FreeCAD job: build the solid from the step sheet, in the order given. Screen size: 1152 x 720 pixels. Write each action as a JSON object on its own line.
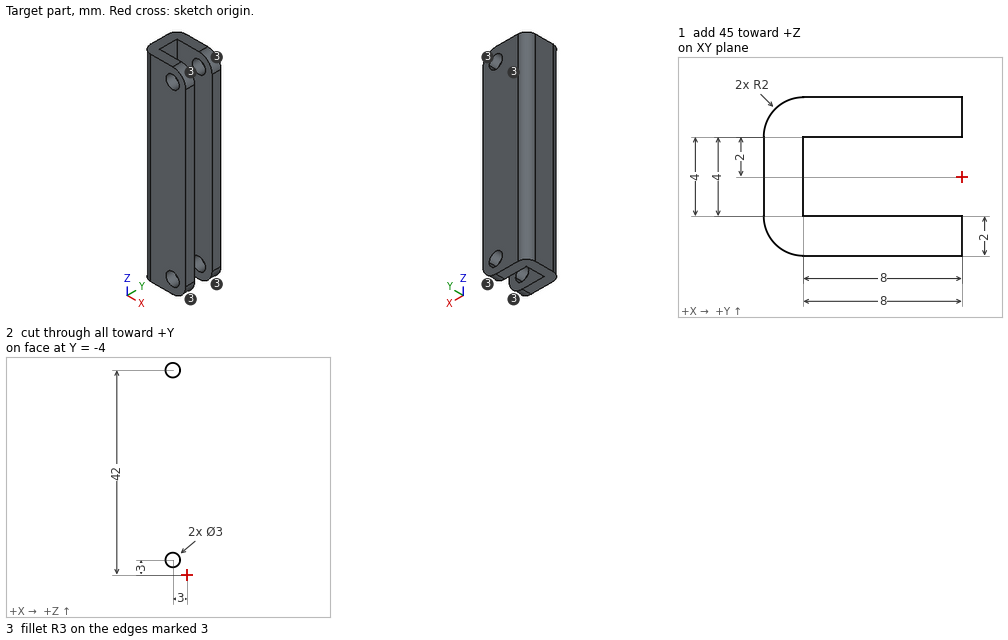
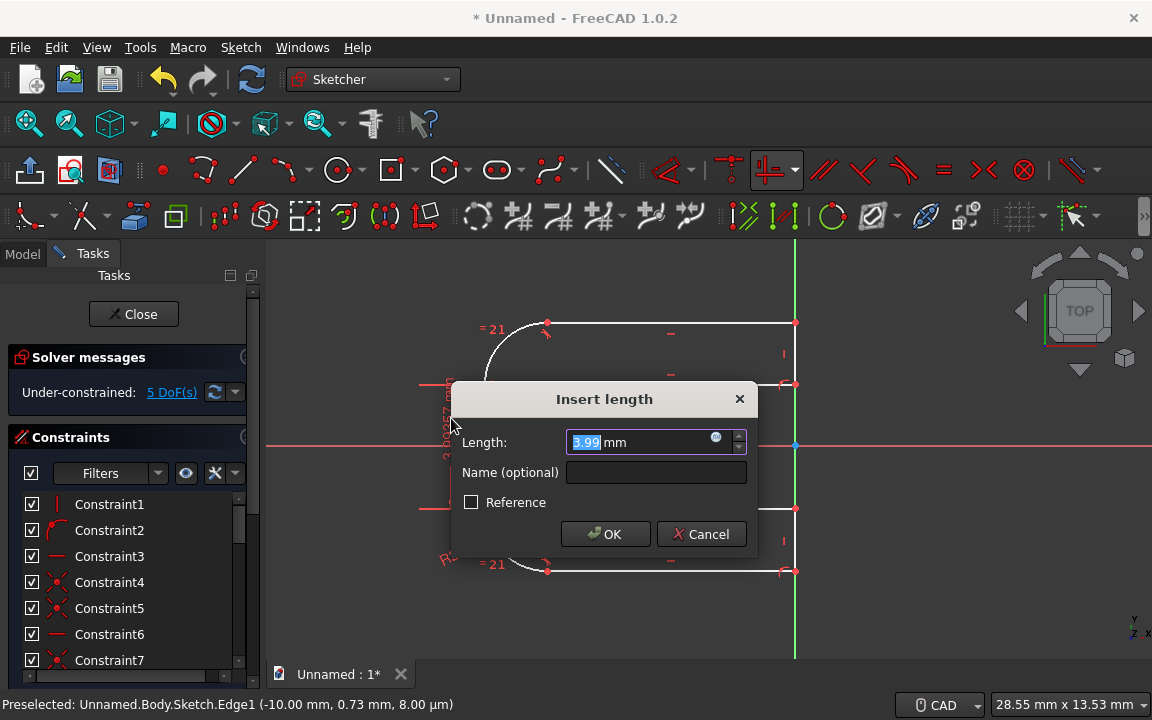
{"action": "type", "text": "4"}
{"action": "key", "text": "Return"}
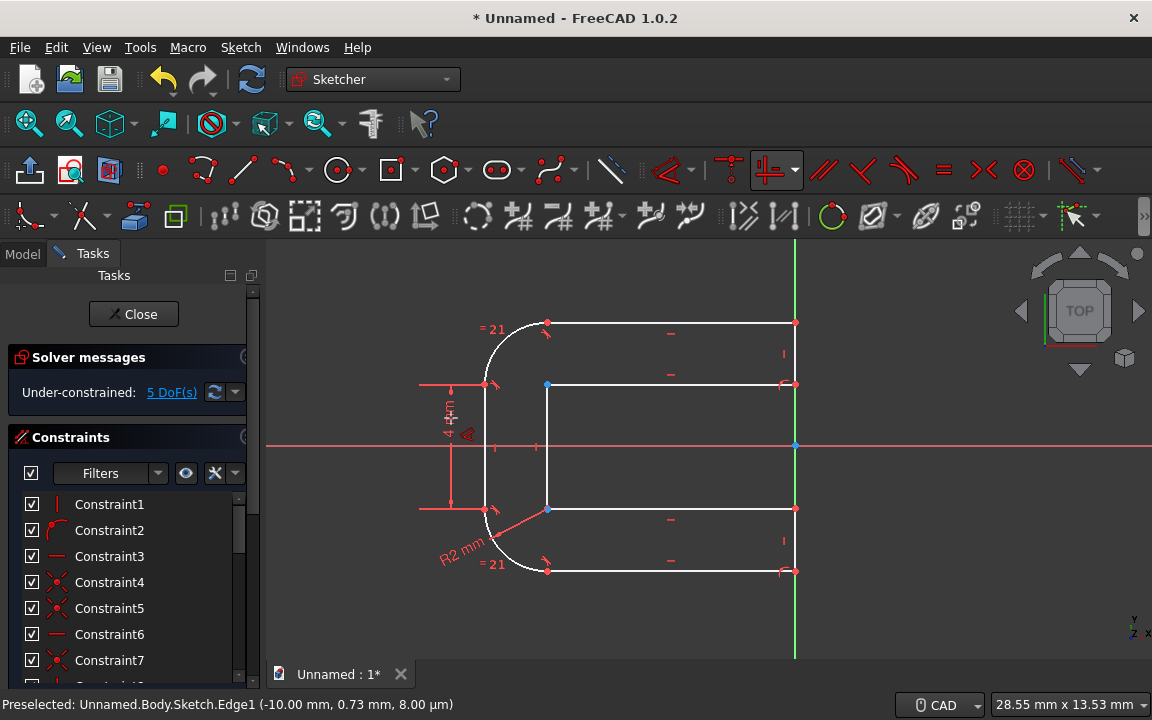
{"action": "left_click", "coordinate": [622, 571]}
{"action": "left_click", "coordinate": [671, 605]}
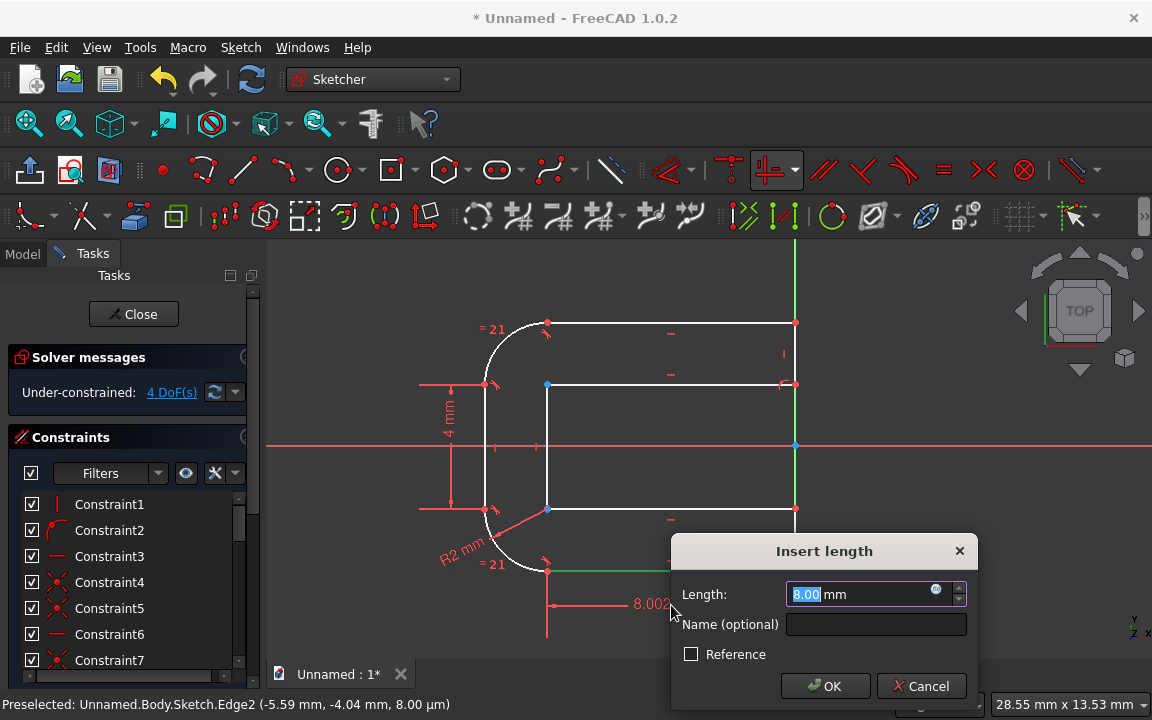
{"action": "type", "text": "8"}
{"action": "key", "text": "Return"}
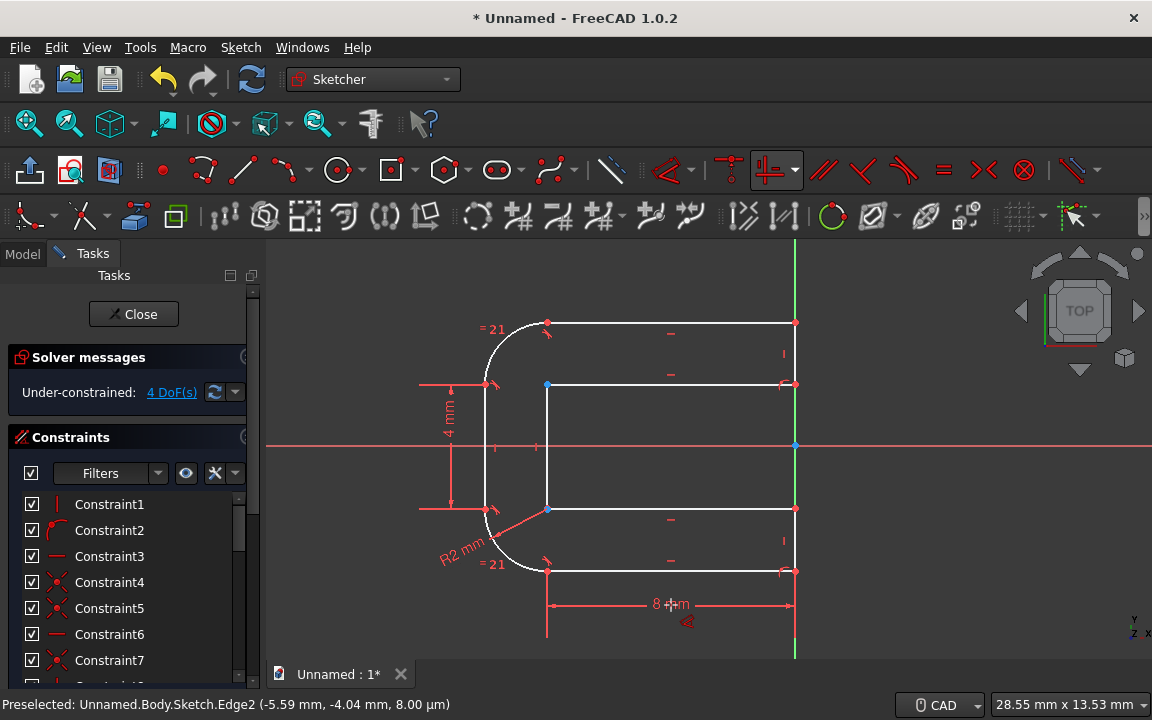
{"action": "left_click", "coordinate": [795, 553]}
{"action": "left_click", "coordinate": [829, 540]}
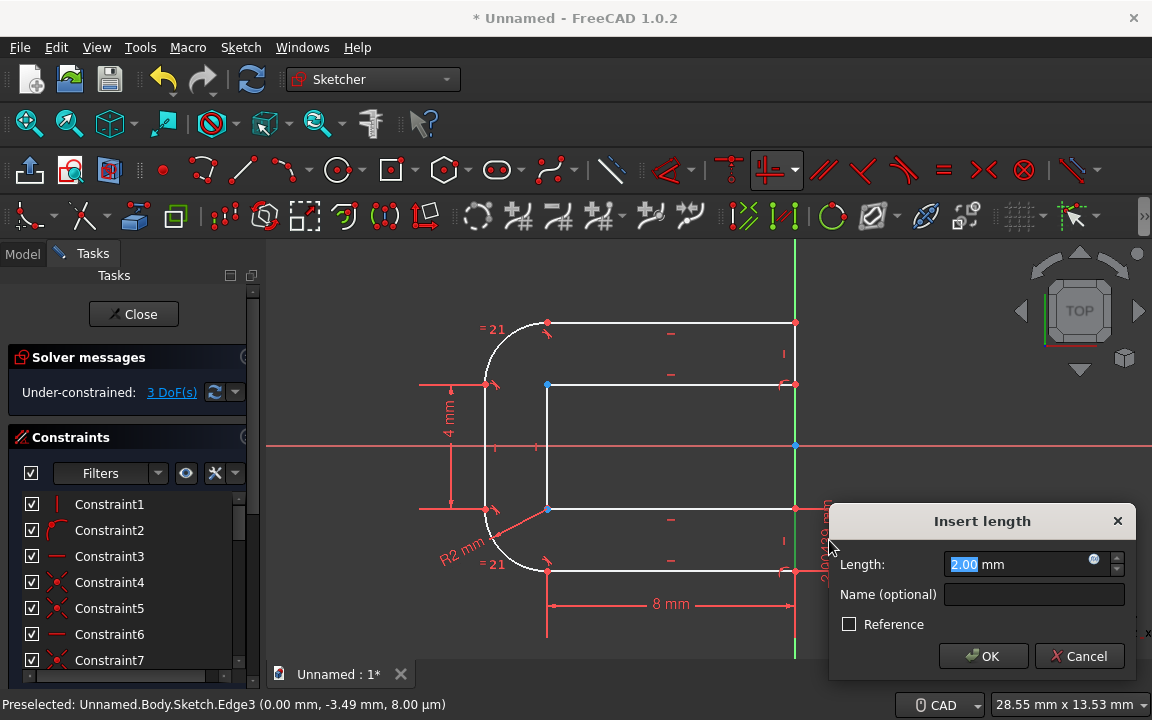
{"action": "type", "text": "2"}
{"action": "key", "text": "Return"}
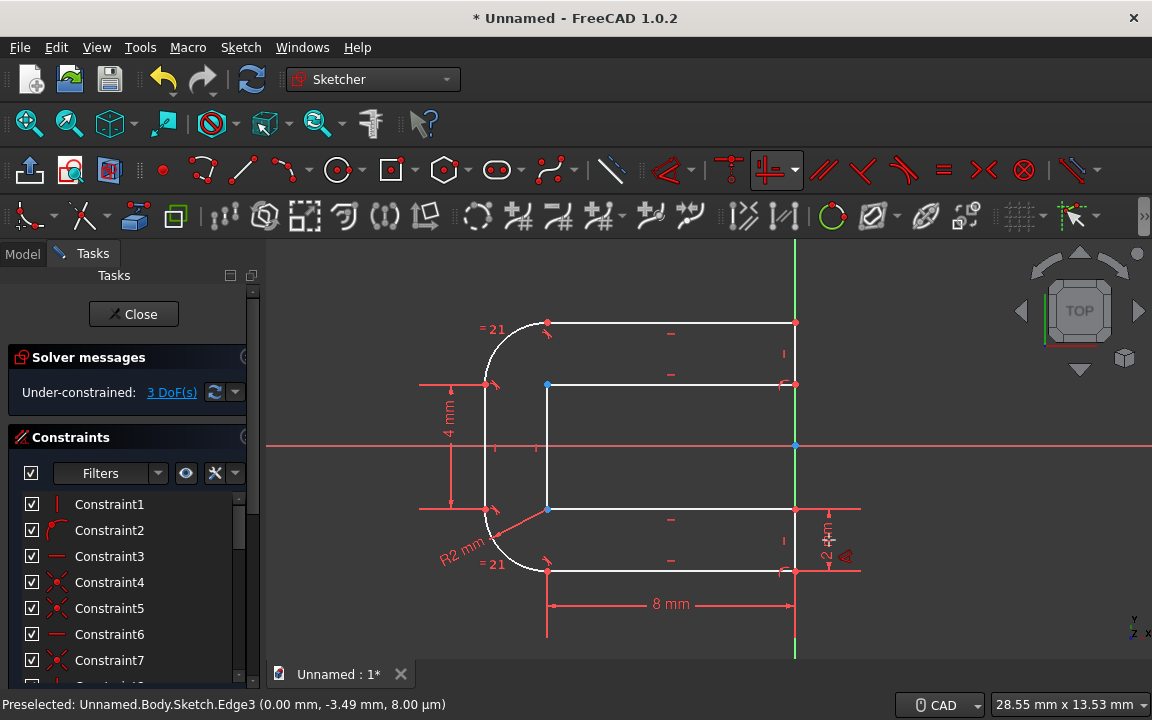
{"action": "left_click", "coordinate": [721, 509]}
{"action": "left_click", "coordinate": [671, 543]}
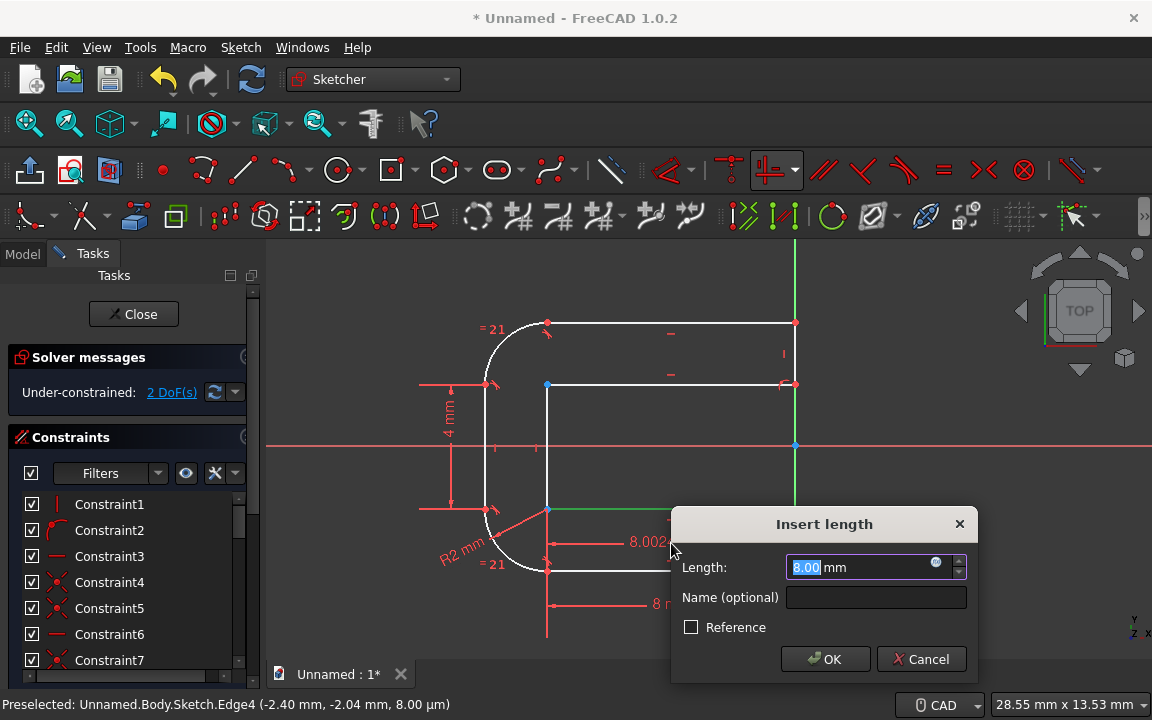
{"action": "type", "text": "8"}
{"action": "key", "text": "Return"}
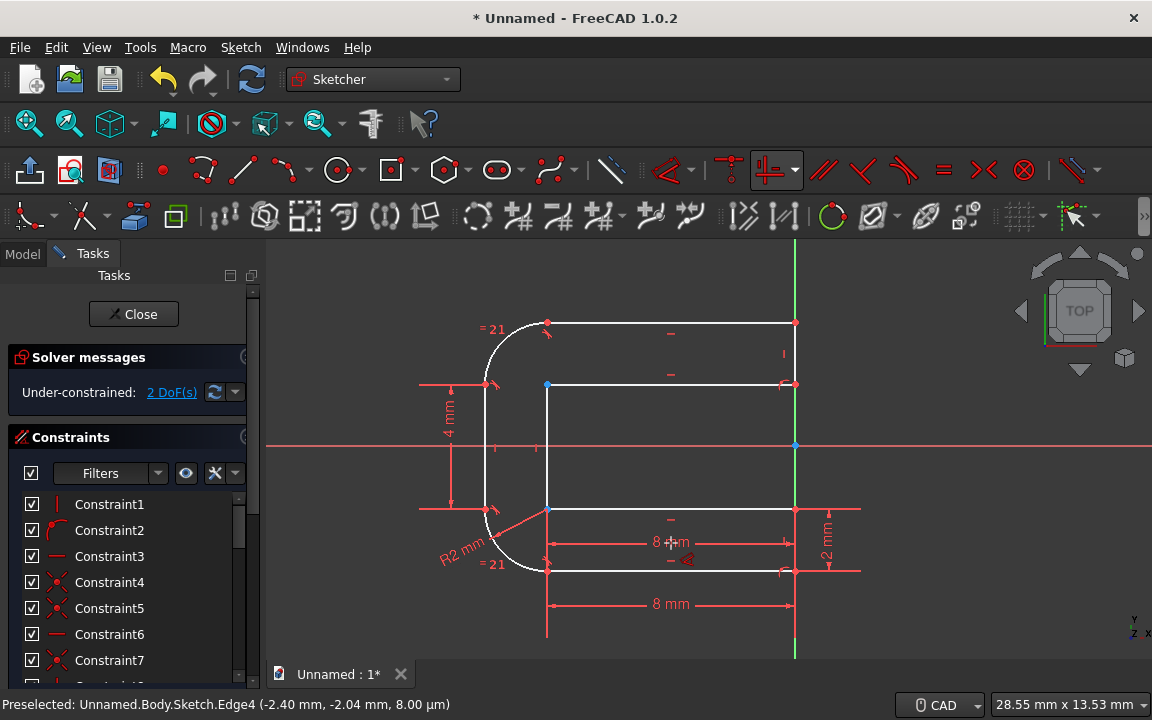
{"action": "left_click", "coordinate": [547, 472]}
{"action": "left_click", "coordinate": [513, 476]}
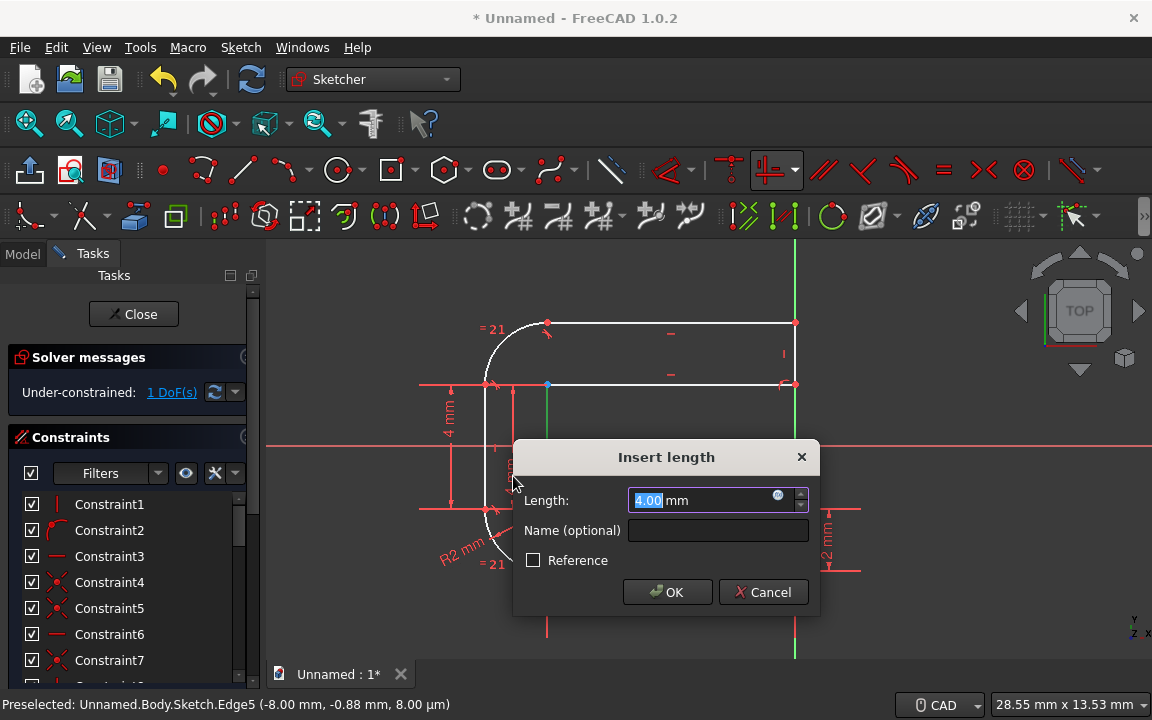
{"action": "type", "text": "4"}
{"action": "key", "text": "Return"}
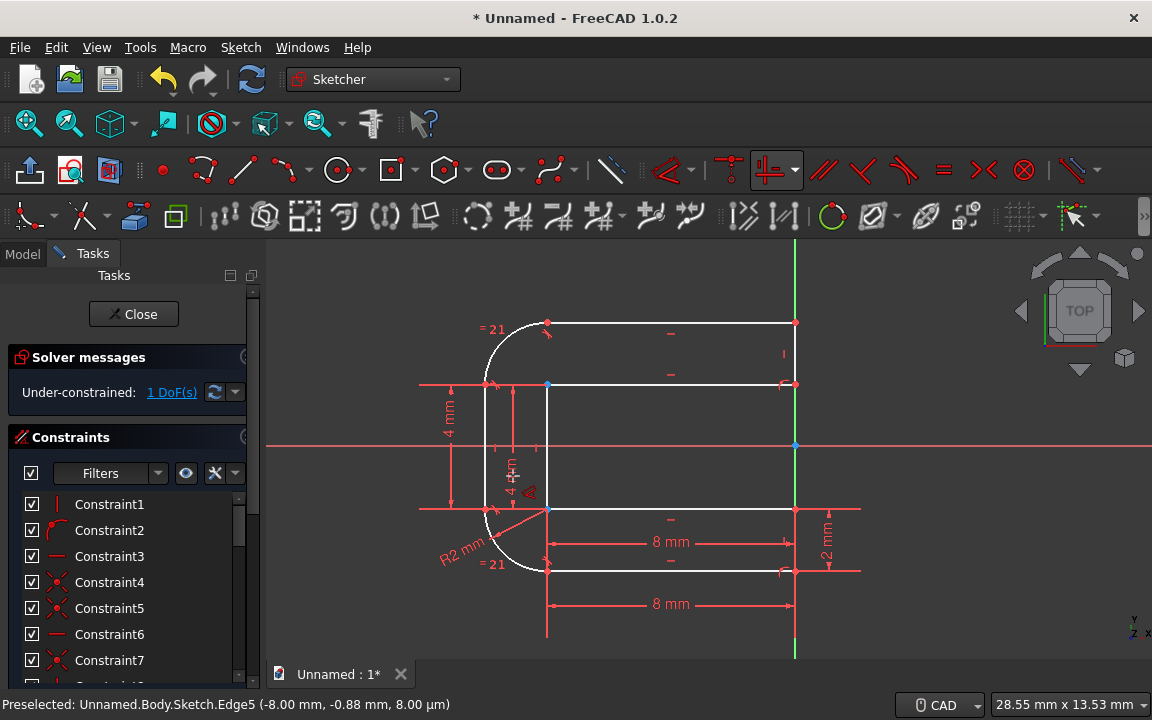
{"action": "left_click", "coordinate": [485, 385]}
{"action": "left_click", "coordinate": [829, 415]}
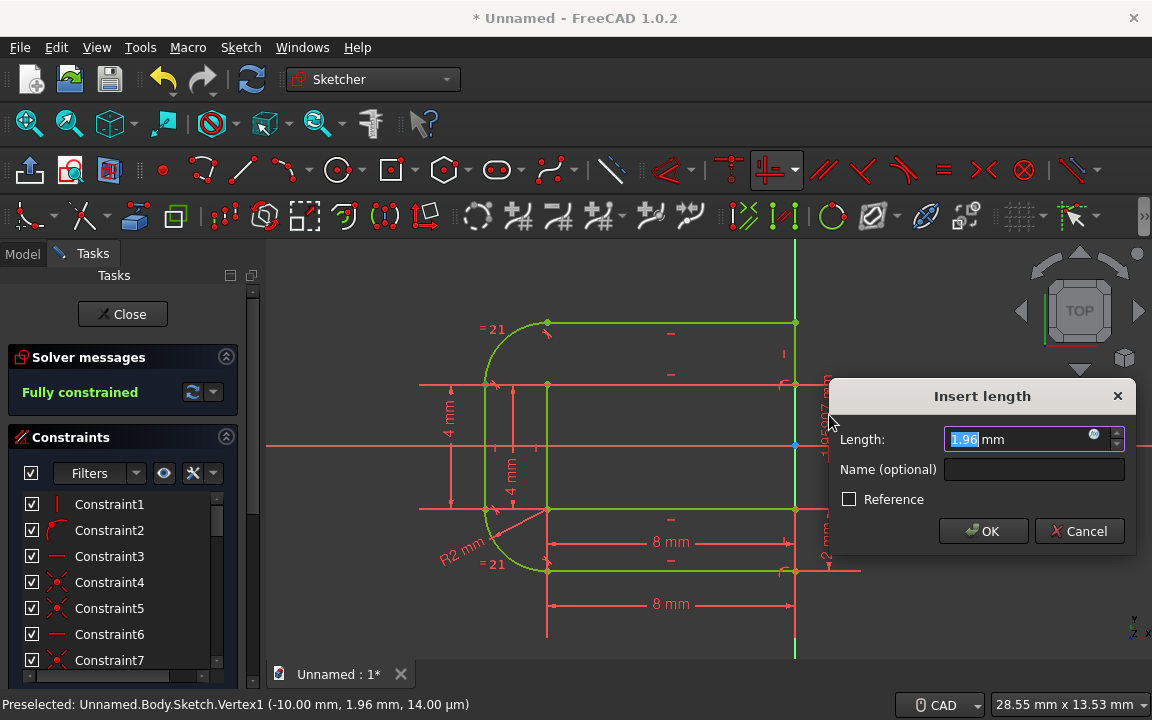
{"action": "type", "text": "2"}
{"action": "key", "text": "Return"}
{"action": "key", "text": "Escape"}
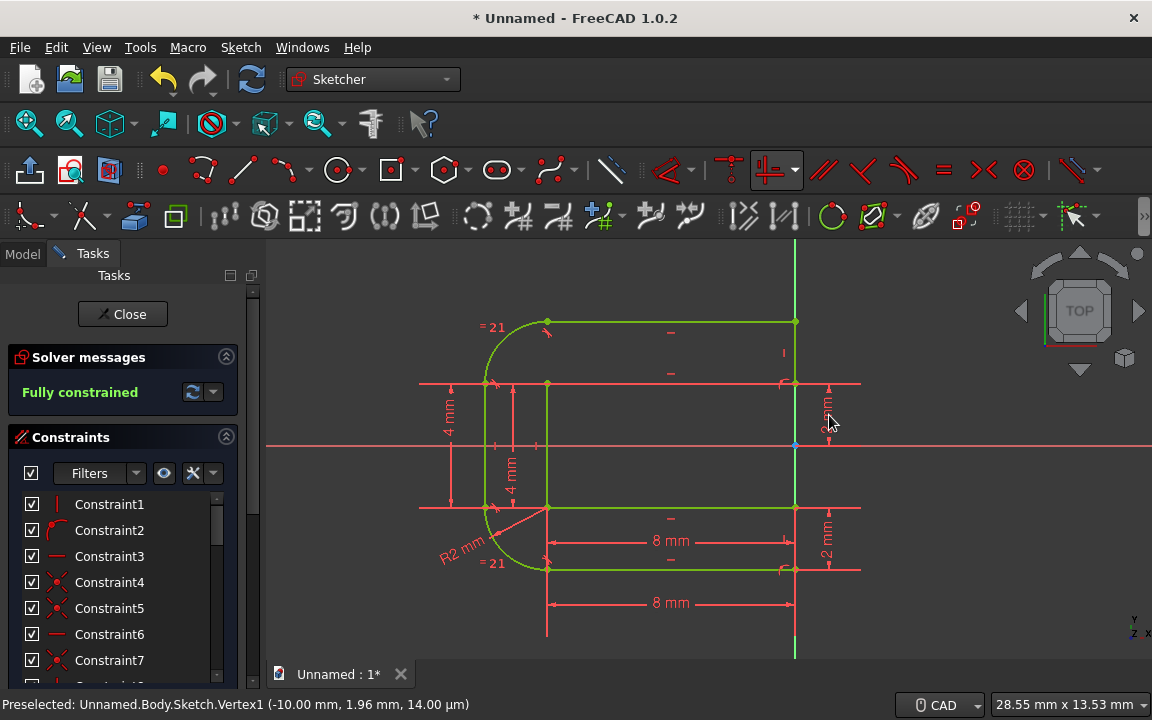
{"action": "left_click", "coordinate": [123, 314]}